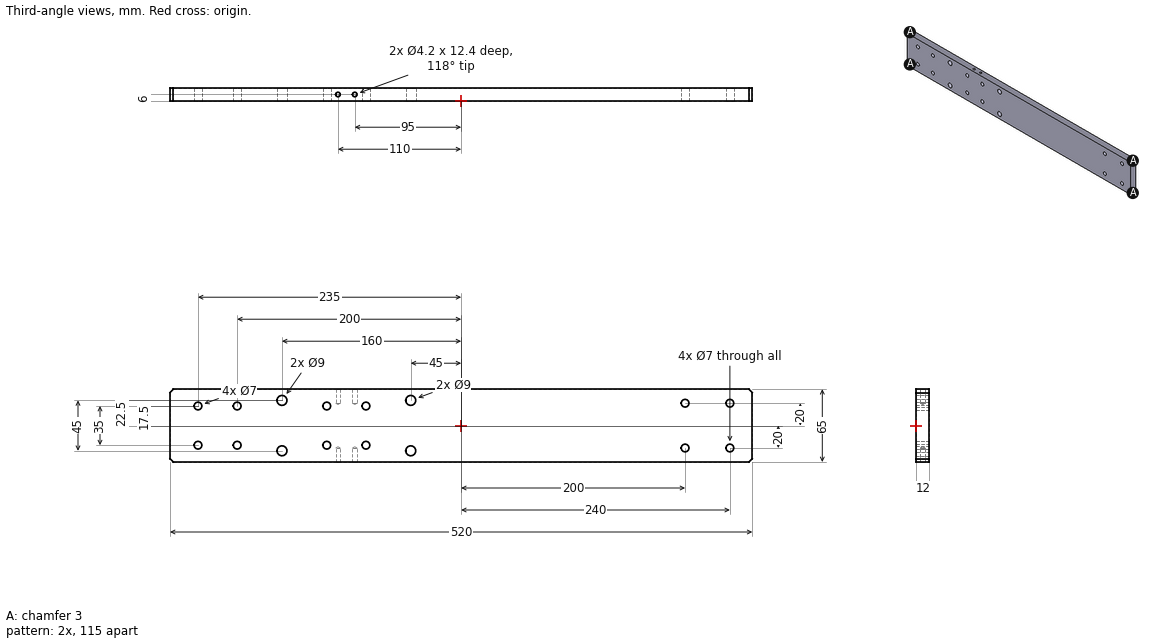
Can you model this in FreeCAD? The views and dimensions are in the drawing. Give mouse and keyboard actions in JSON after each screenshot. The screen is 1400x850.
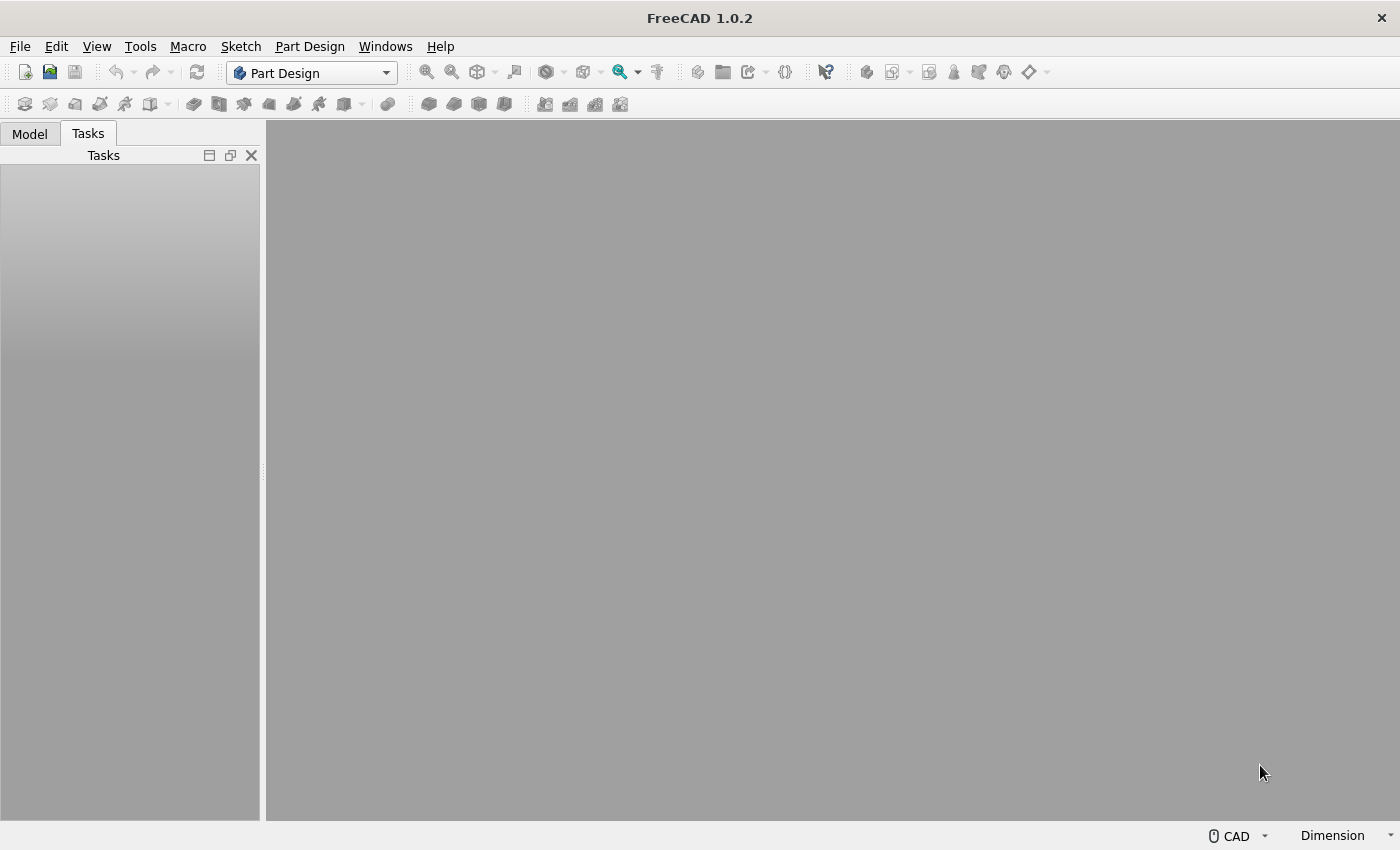
{"action": "left_click", "coordinate": [25, 72]}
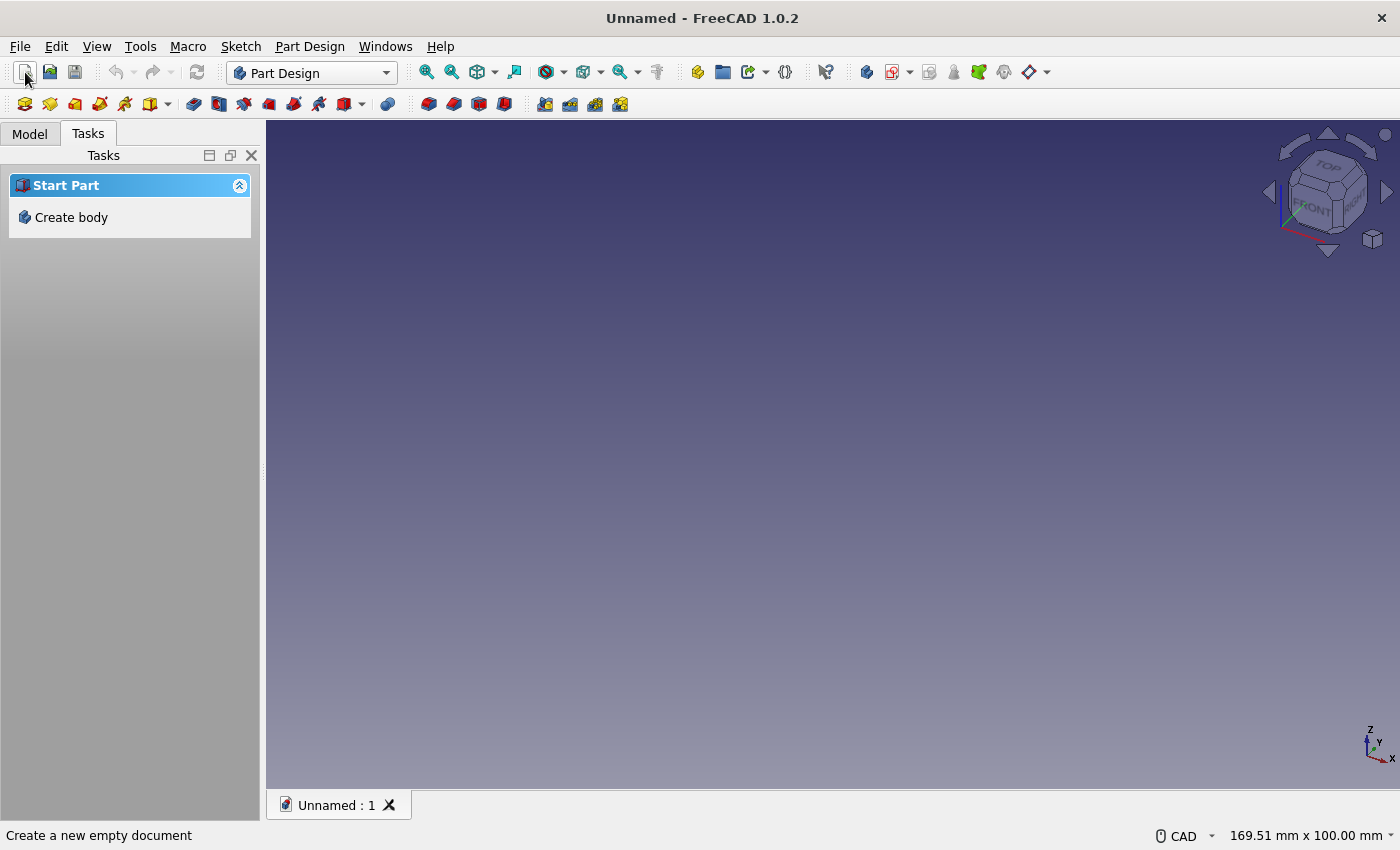
{"action": "left_click", "coordinate": [892, 72]}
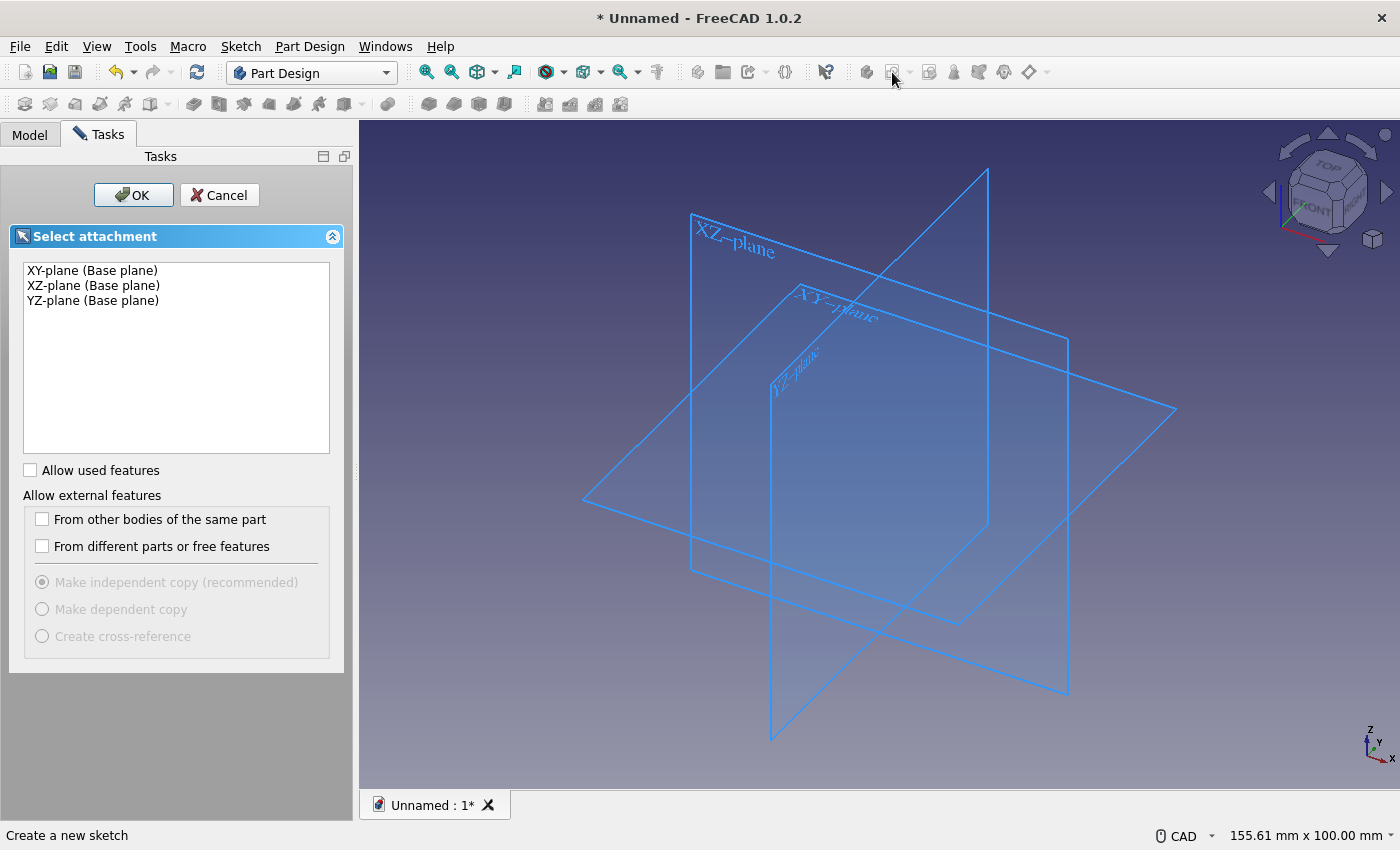
{"action": "left_click", "coordinate": [84, 286]}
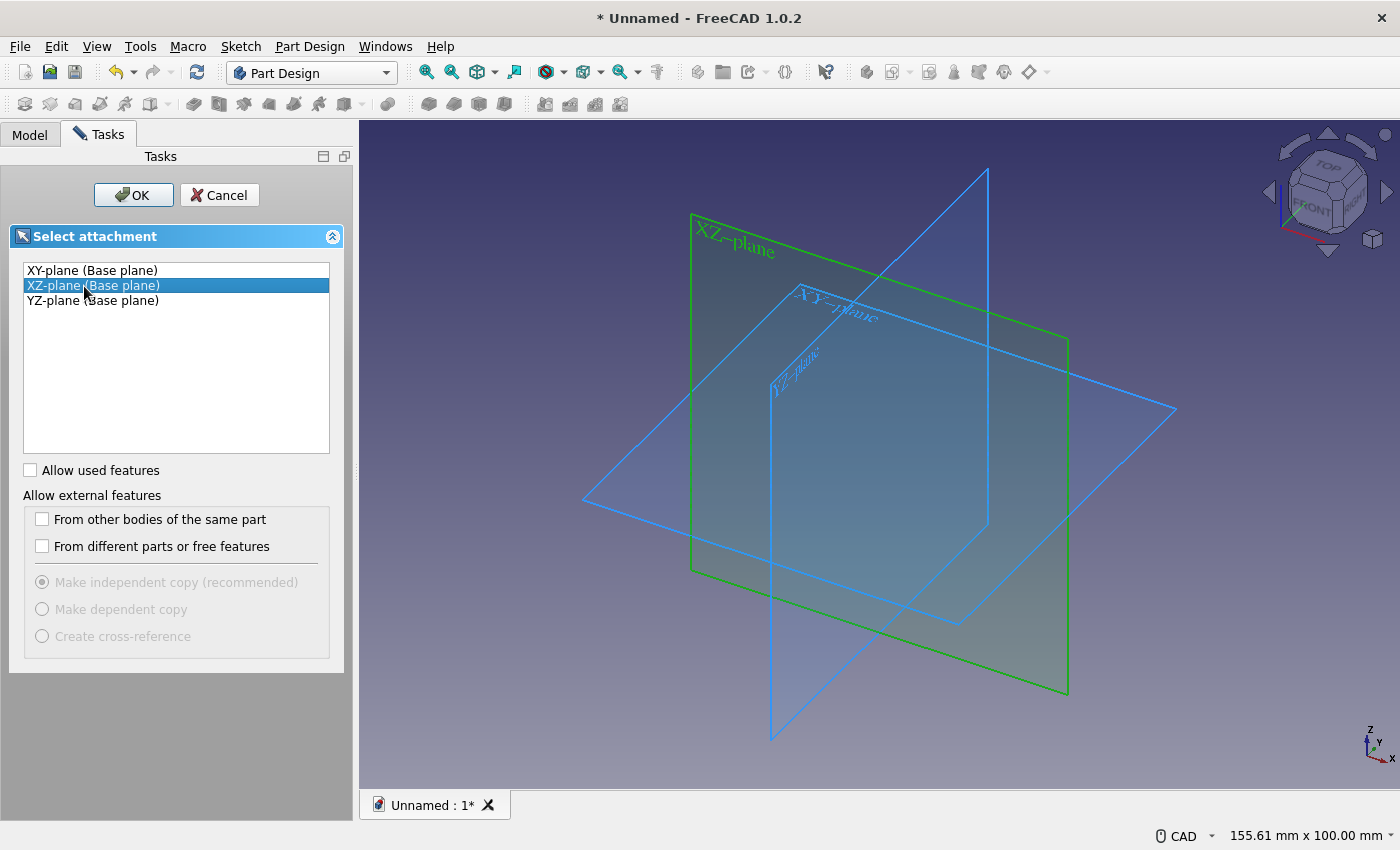
{"action": "left_click", "coordinate": [134, 195]}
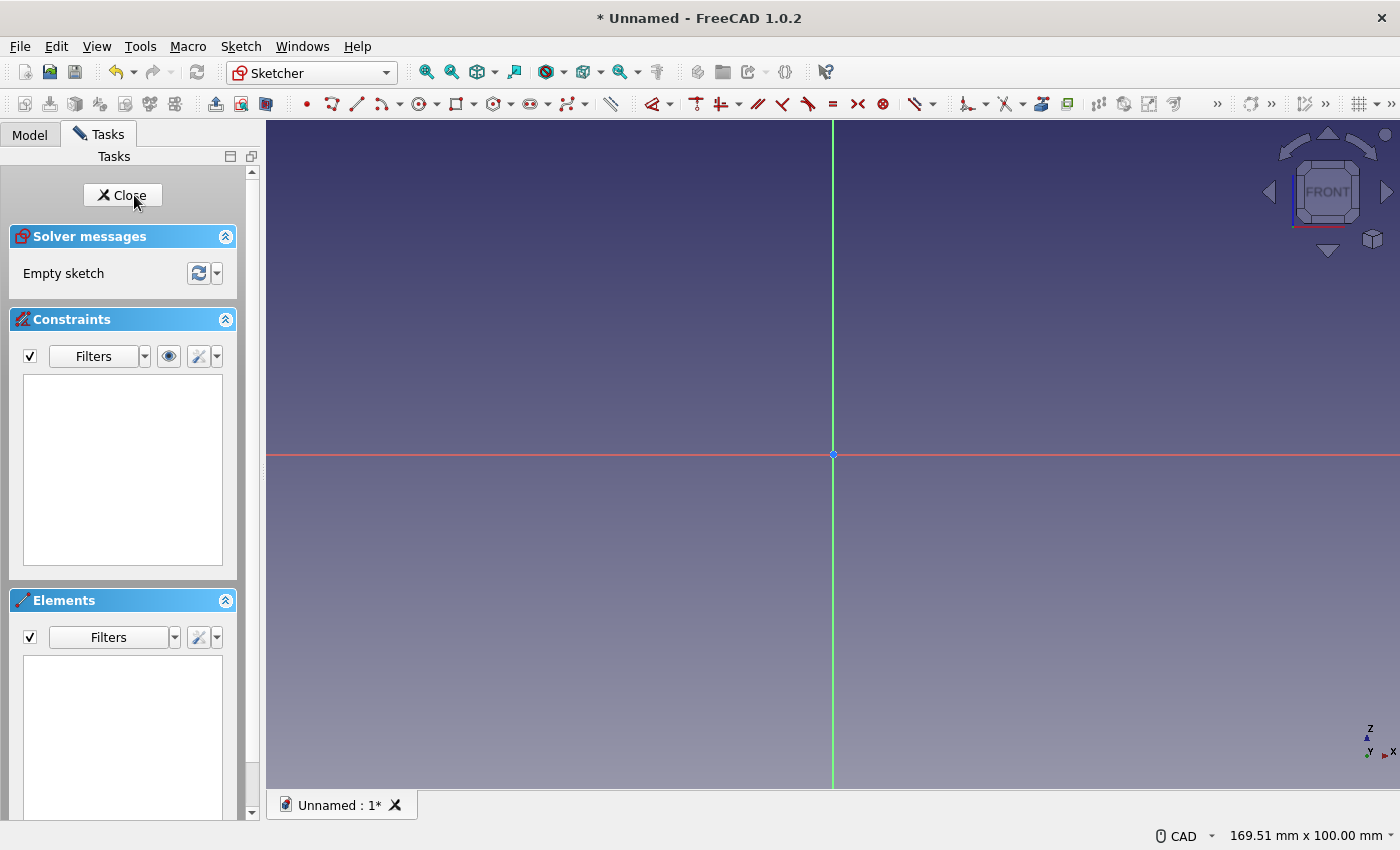
{"action": "scroll", "coordinate": [747, 454], "scroll_direction": "down", "scroll_amount": 8}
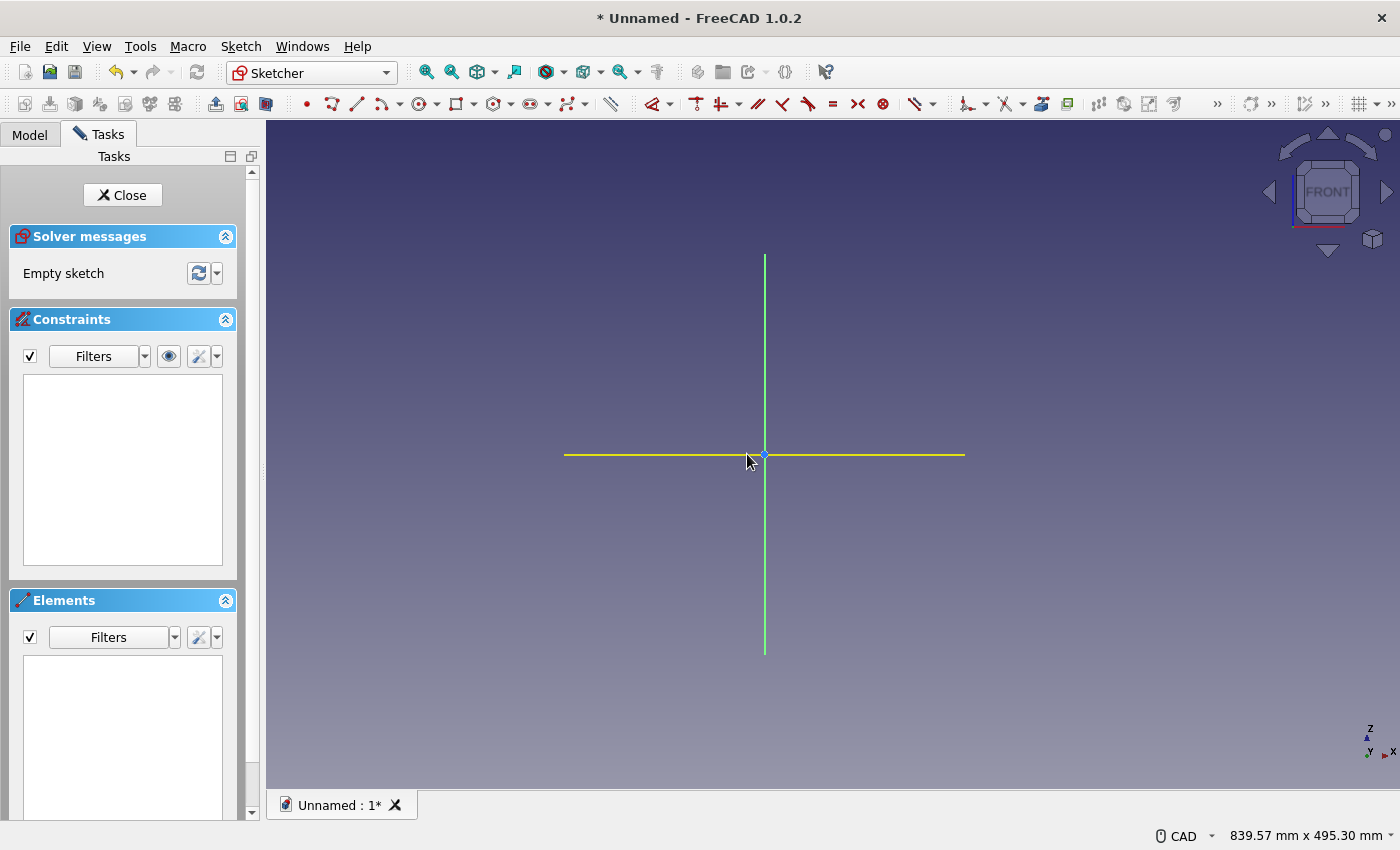
{"action": "left_click", "coordinate": [474, 104]}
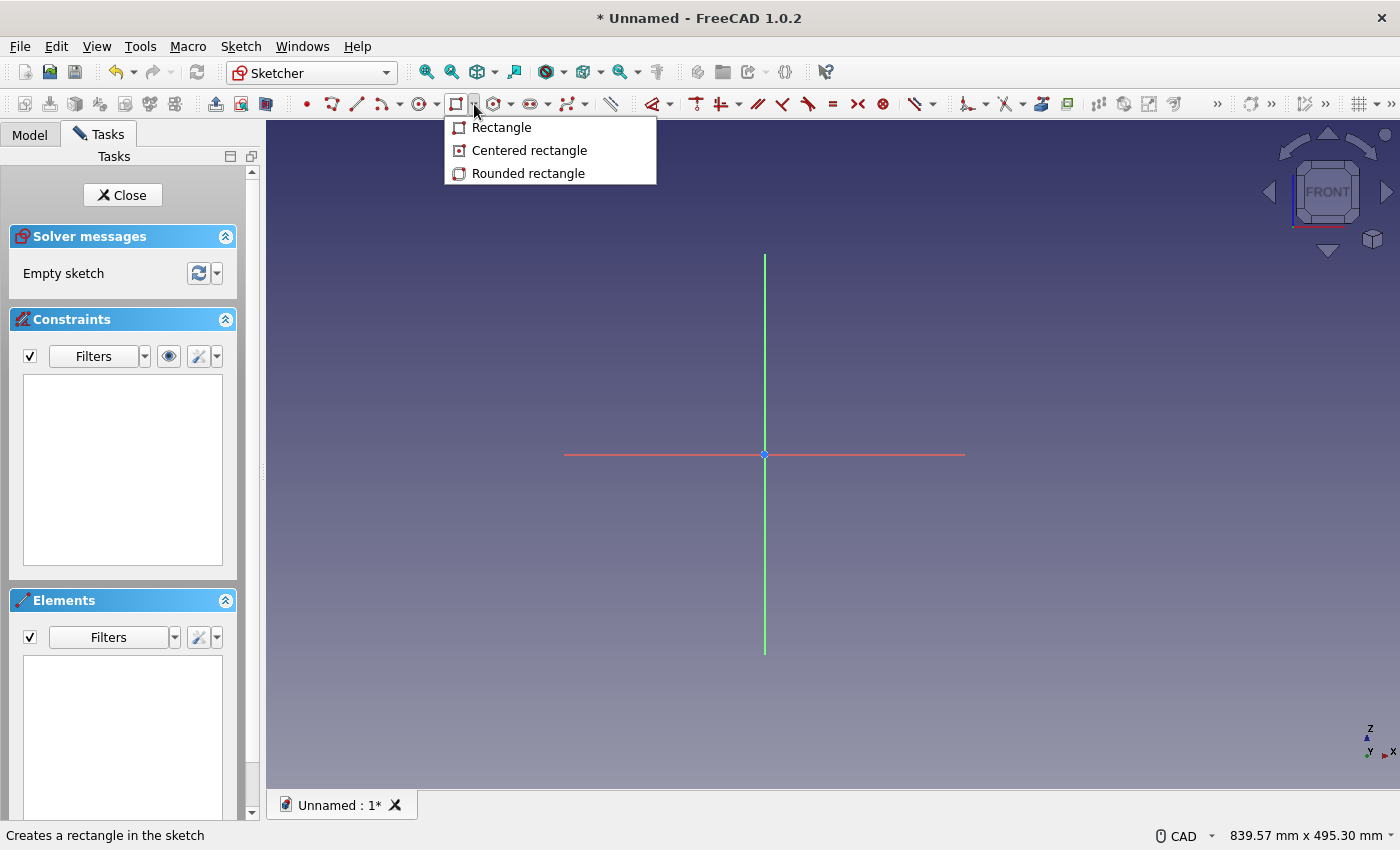
{"action": "left_click", "coordinate": [550, 150]}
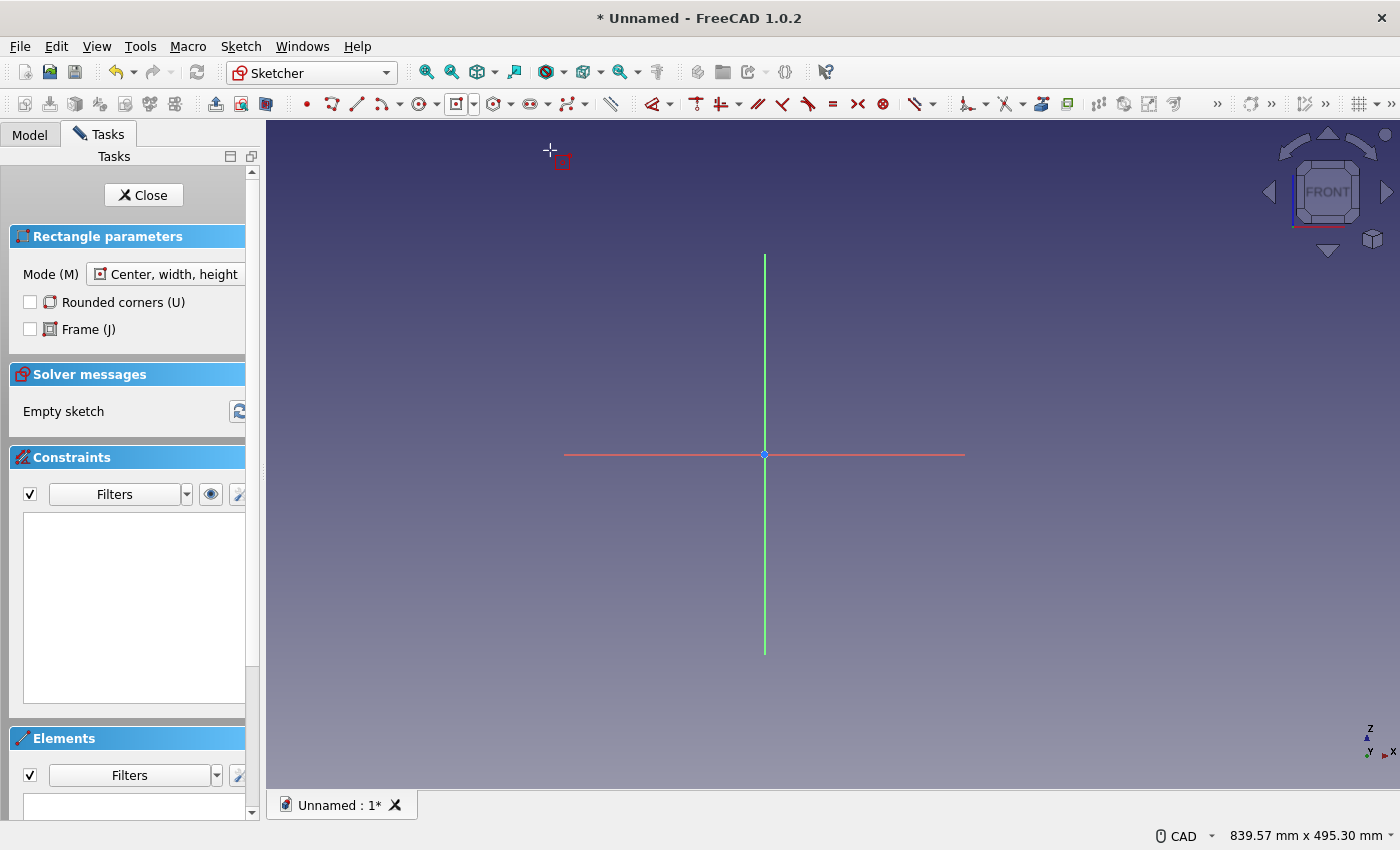
{"action": "left_click", "coordinate": [765, 454]}
{"action": "left_click", "coordinate": [1116, 411]}
{"action": "key", "text": "Escape"}